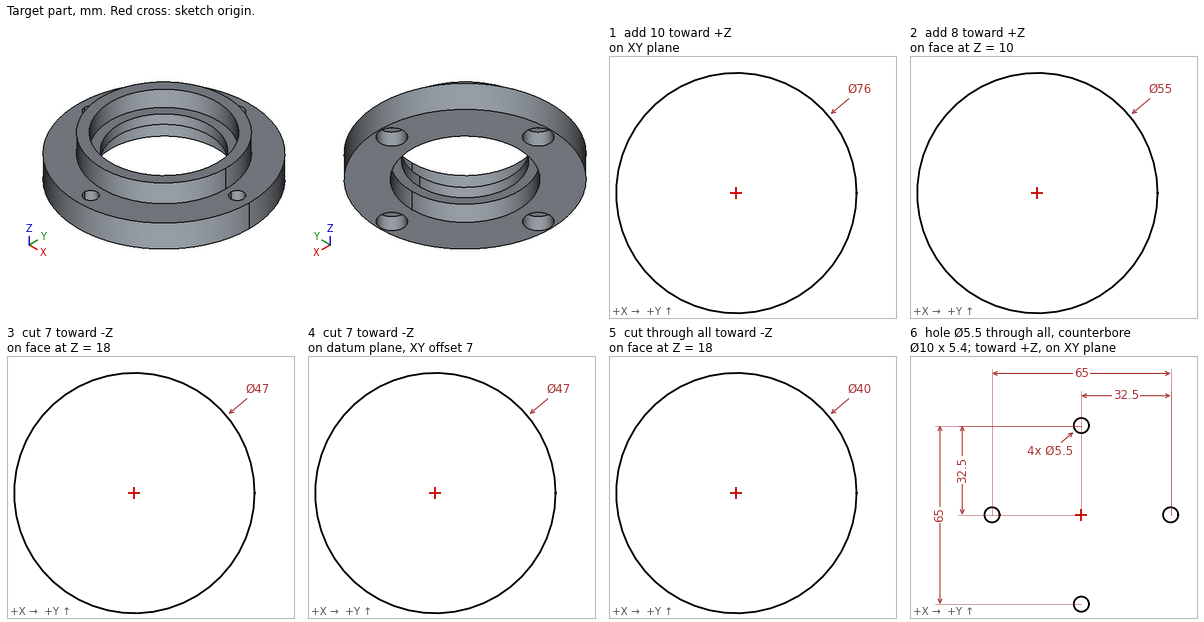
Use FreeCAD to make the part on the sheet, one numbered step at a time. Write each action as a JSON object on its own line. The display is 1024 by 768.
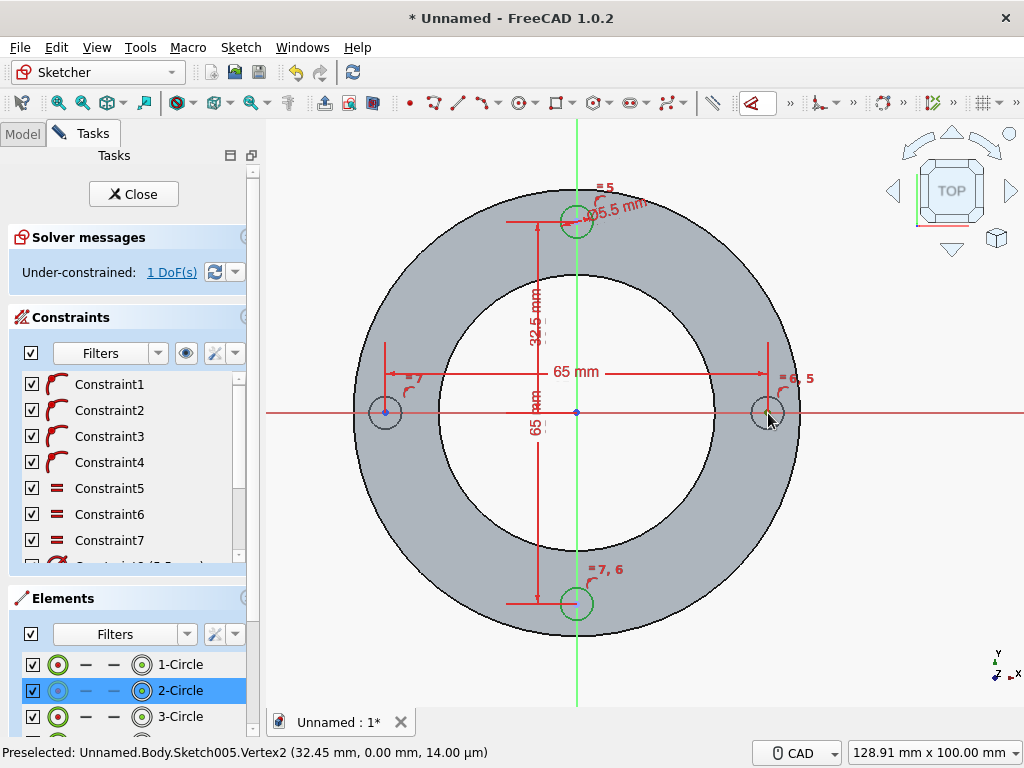
{"action": "key", "text": "l"}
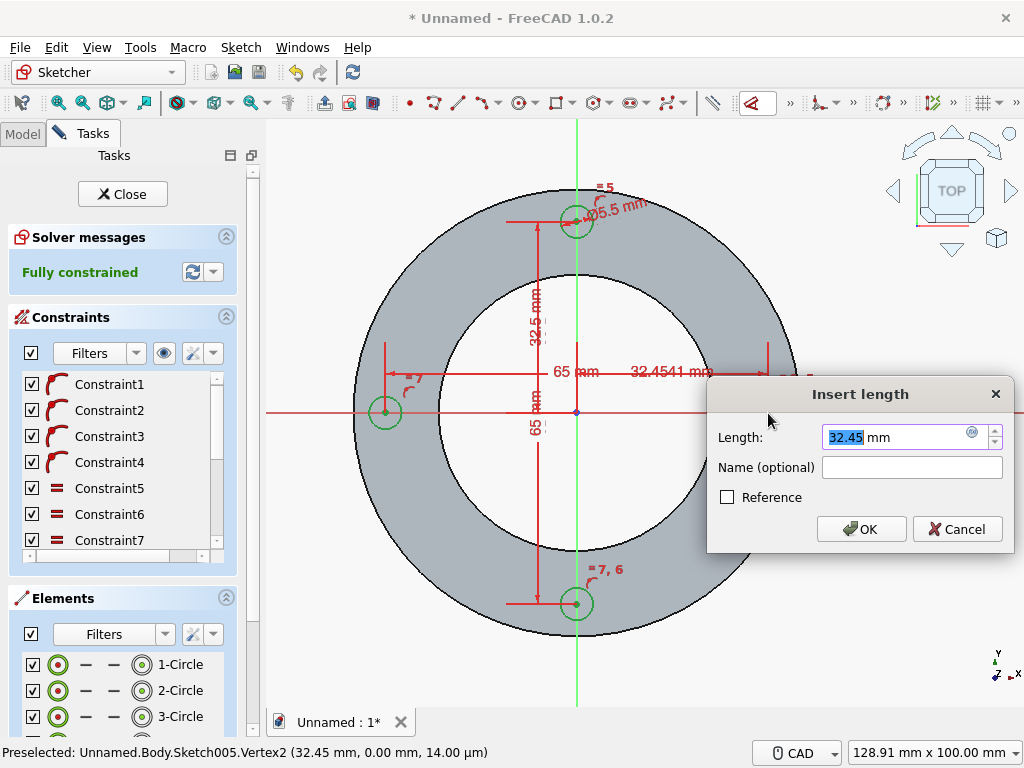
{"action": "type", "text": "32.5"}
{"action": "key", "text": "Return"}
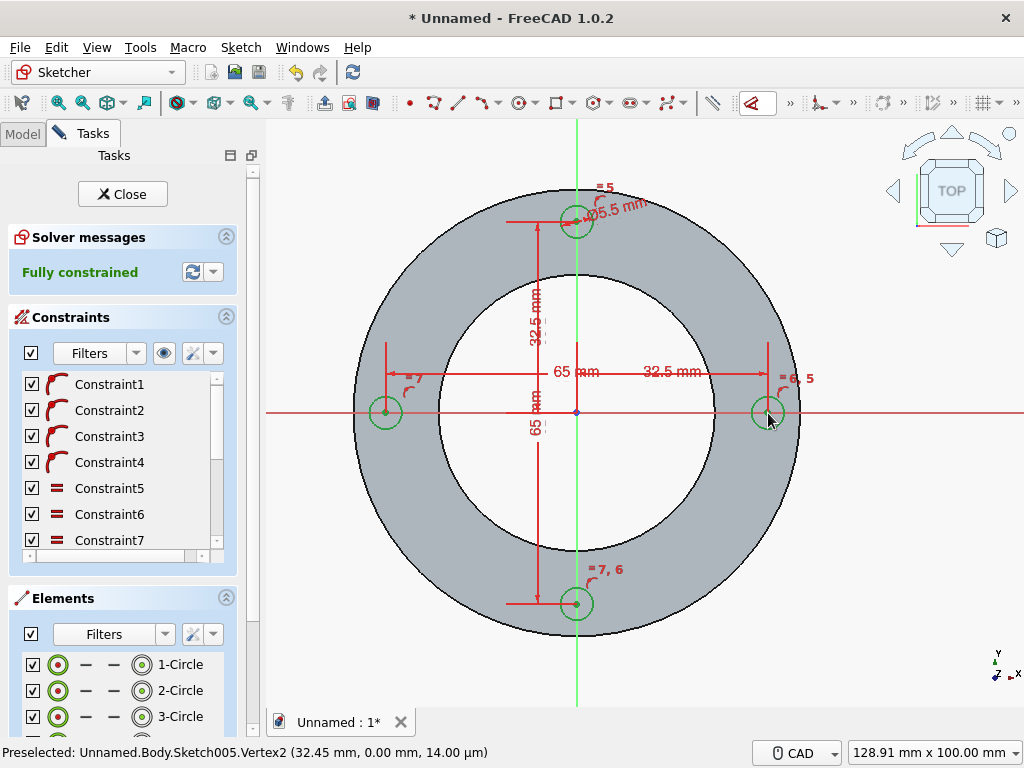
{"action": "left_click", "coordinate": [123, 194]}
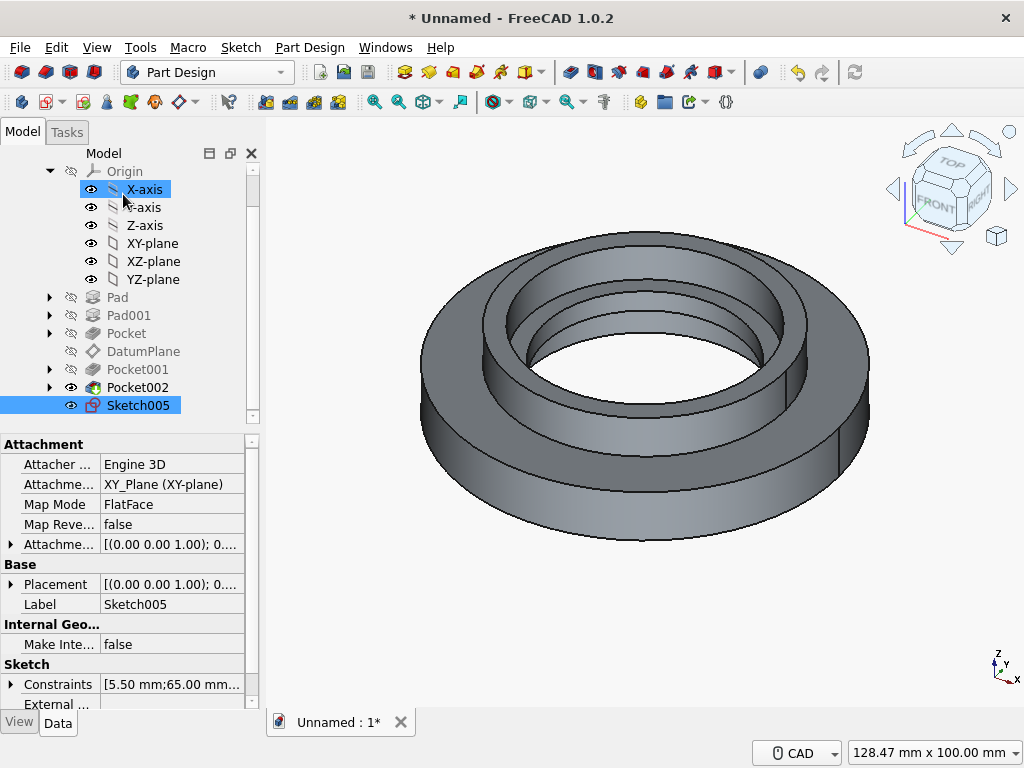
{"action": "left_click", "coordinate": [596, 72]}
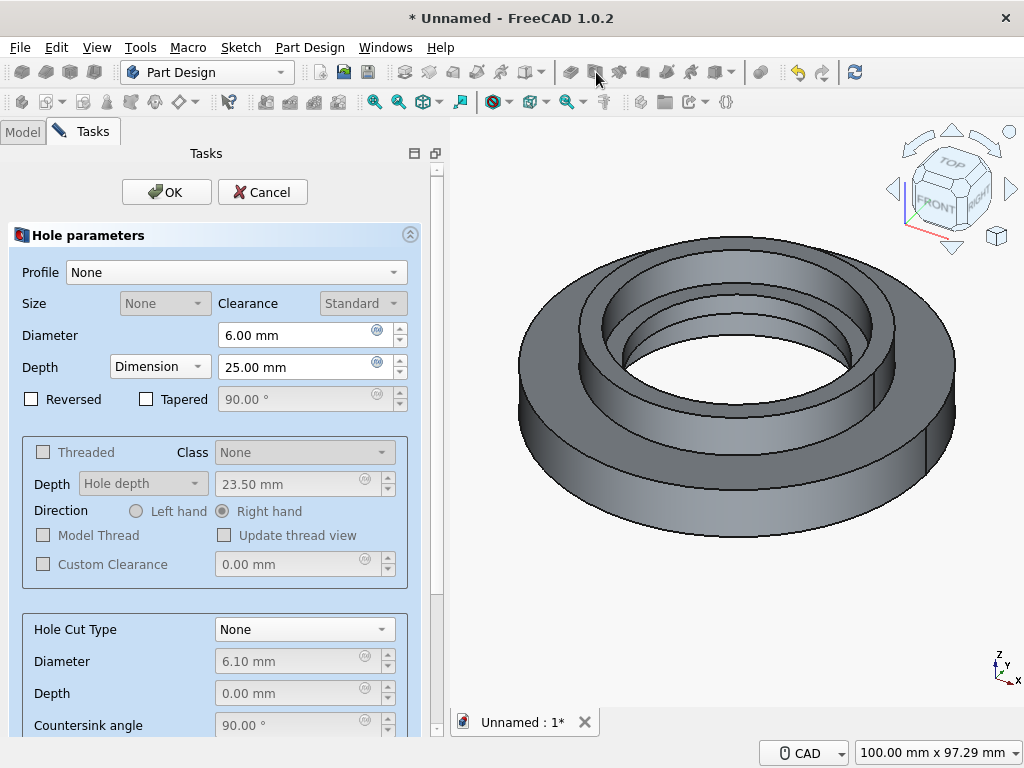
{"action": "triple_click", "coordinate": [305, 335]}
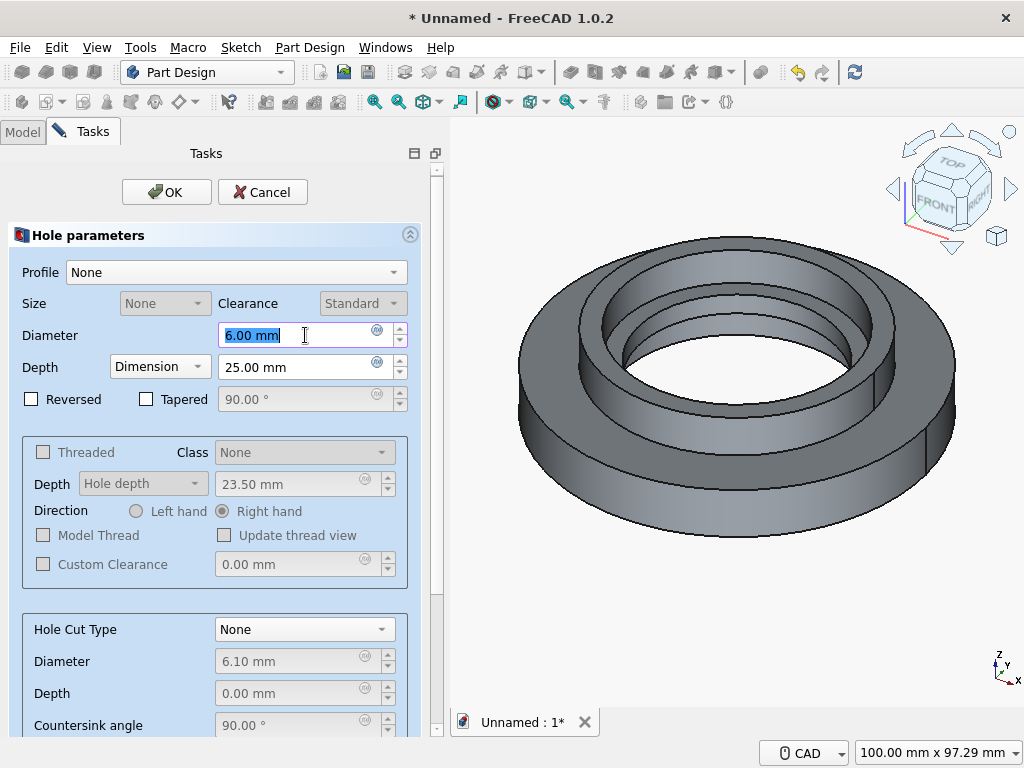
{"action": "type", "text": "5.5"}
{"action": "key", "text": "Tab"}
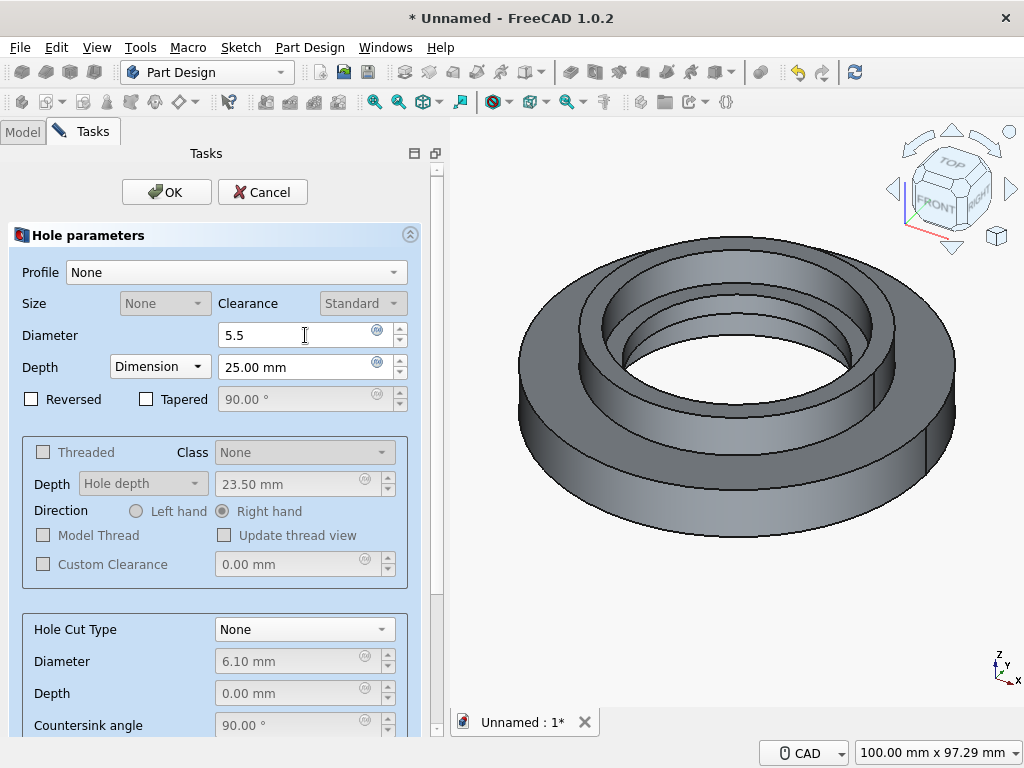
{"action": "left_click", "coordinate": [161, 366]}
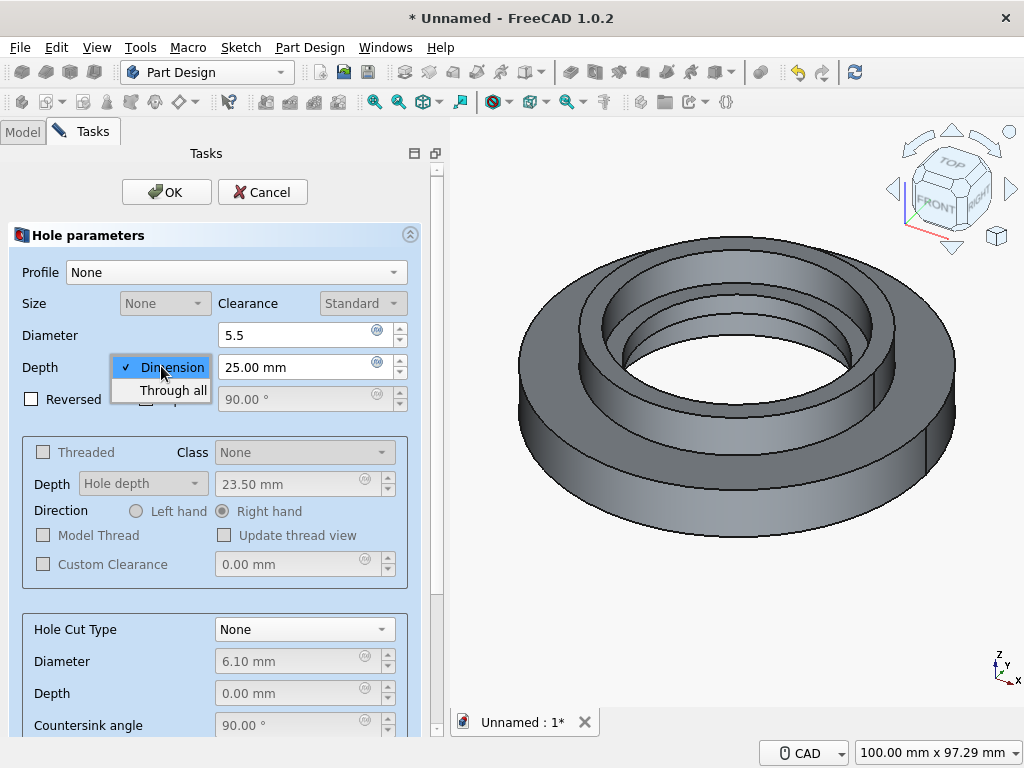
{"action": "left_click", "coordinate": [160, 390]}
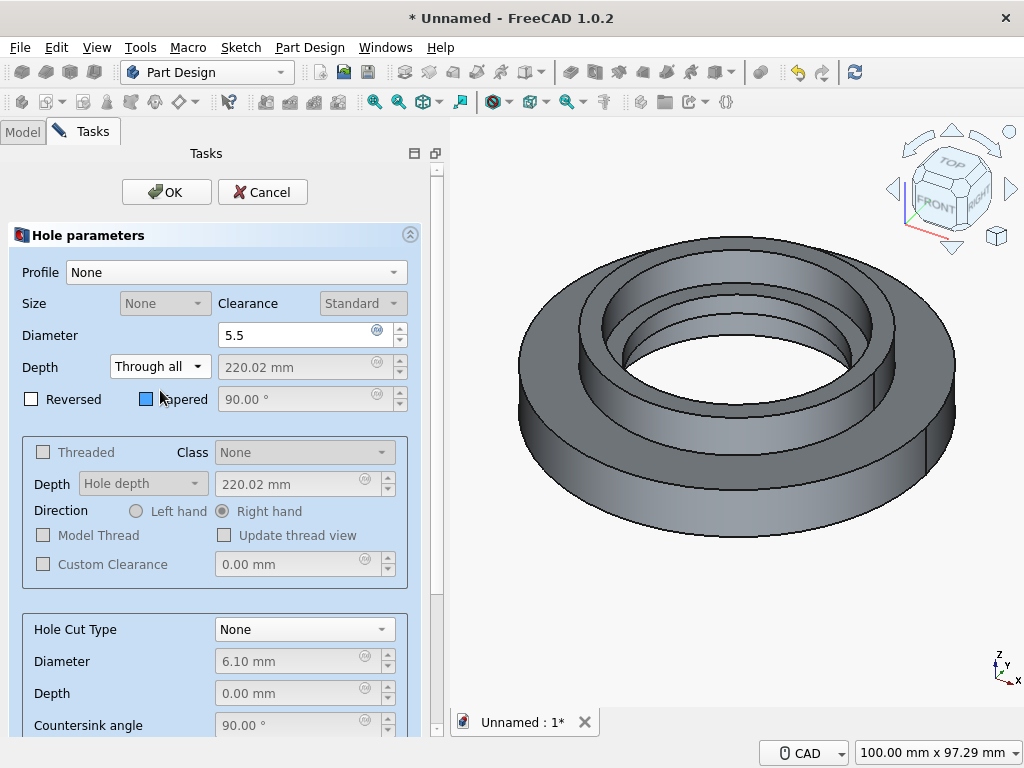
{"action": "left_click", "coordinate": [30, 399]}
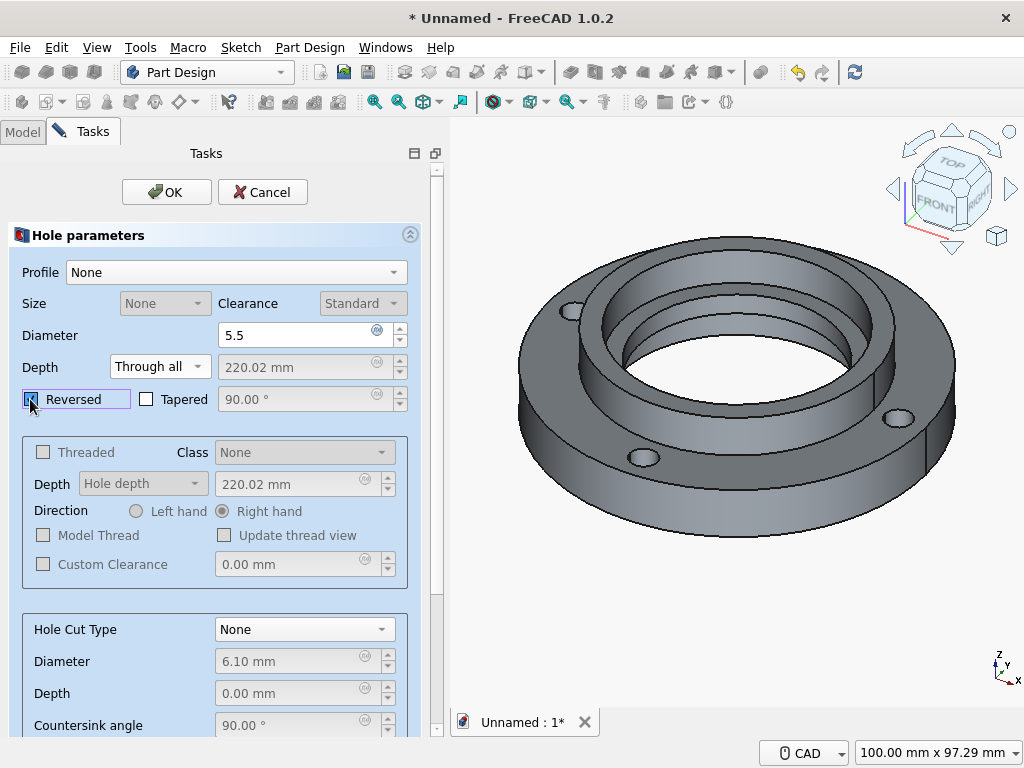
{"action": "left_click", "coordinate": [306, 630]}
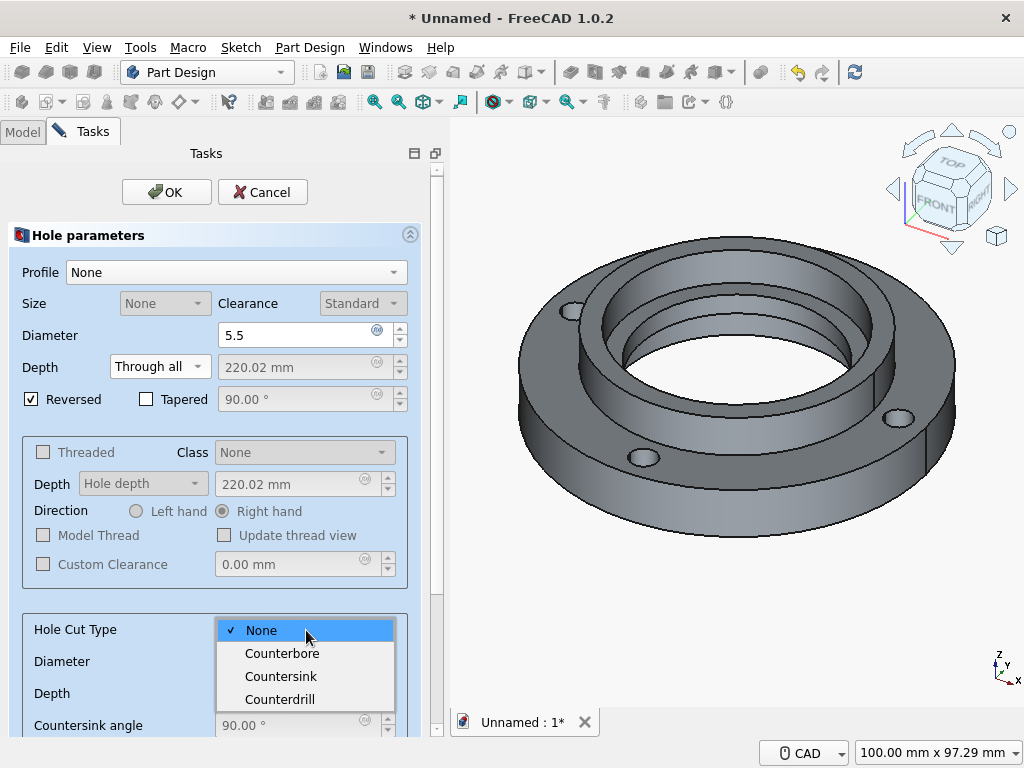
{"action": "left_click", "coordinate": [304, 654]}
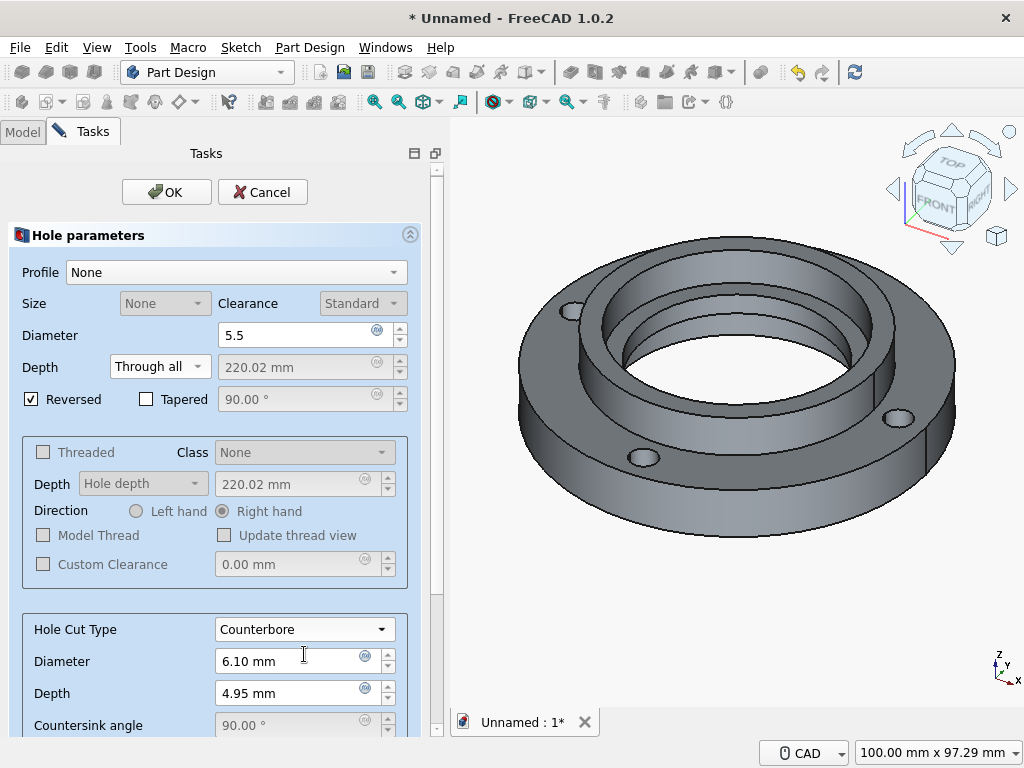
{"action": "triple_click", "coordinate": [298, 661]}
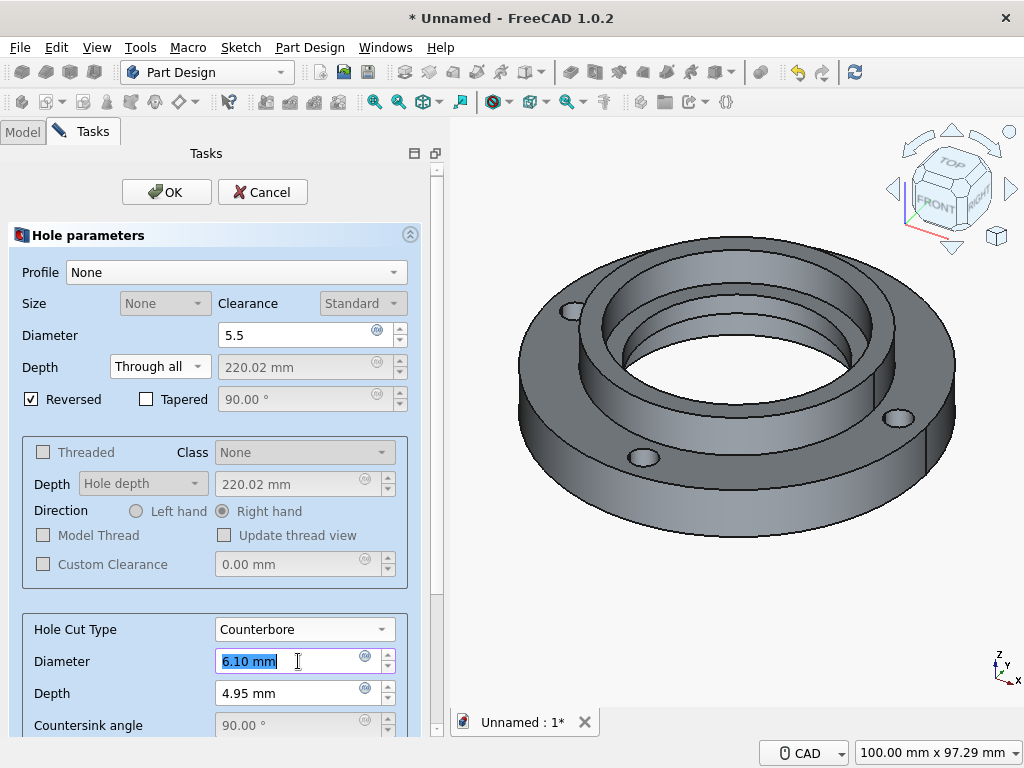
{"action": "type", "text": "10"}
{"action": "key", "text": "Tab"}